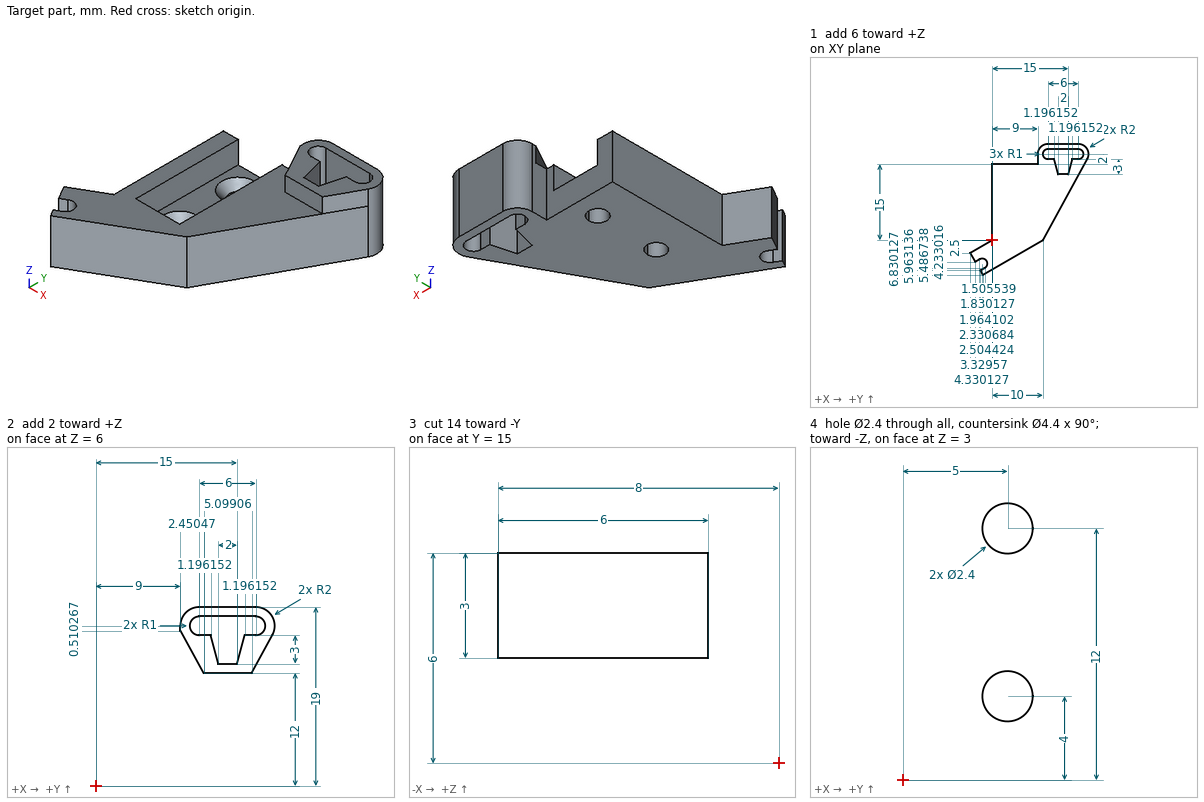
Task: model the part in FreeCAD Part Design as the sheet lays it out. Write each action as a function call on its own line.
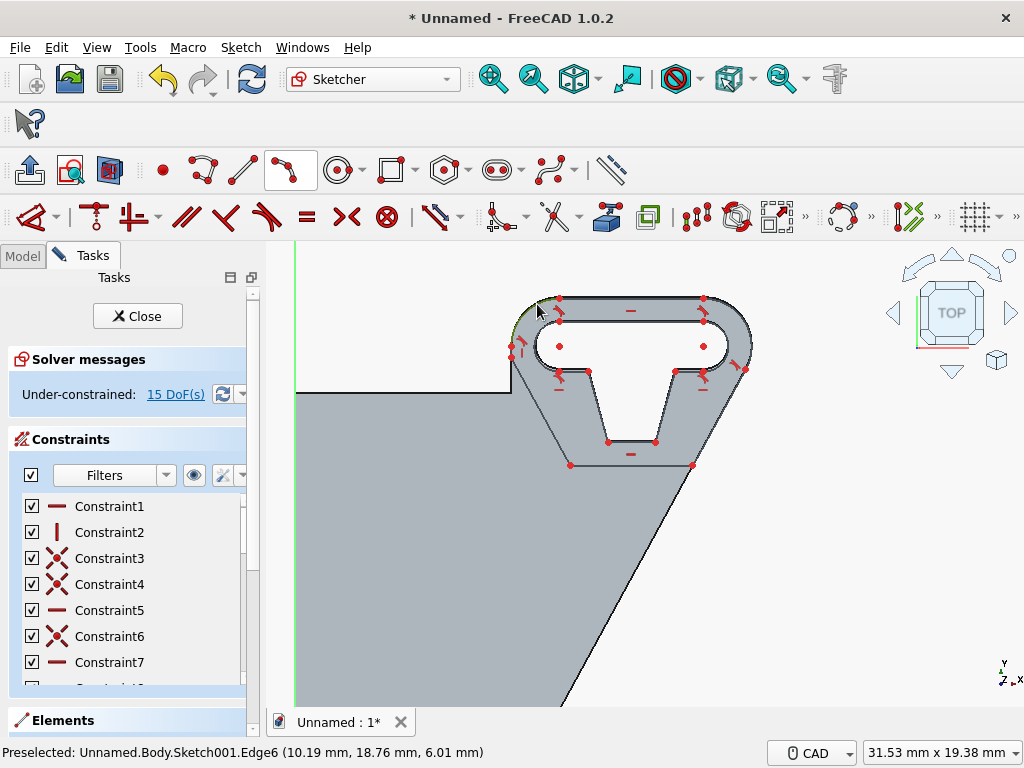
click(751, 341)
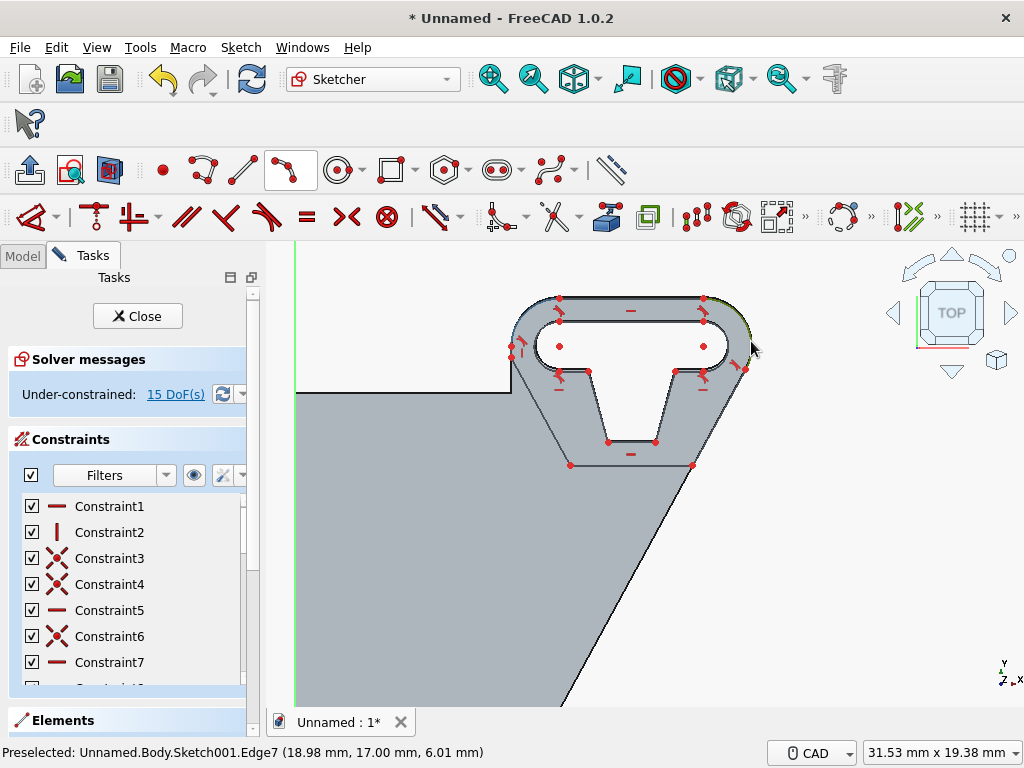
key(e)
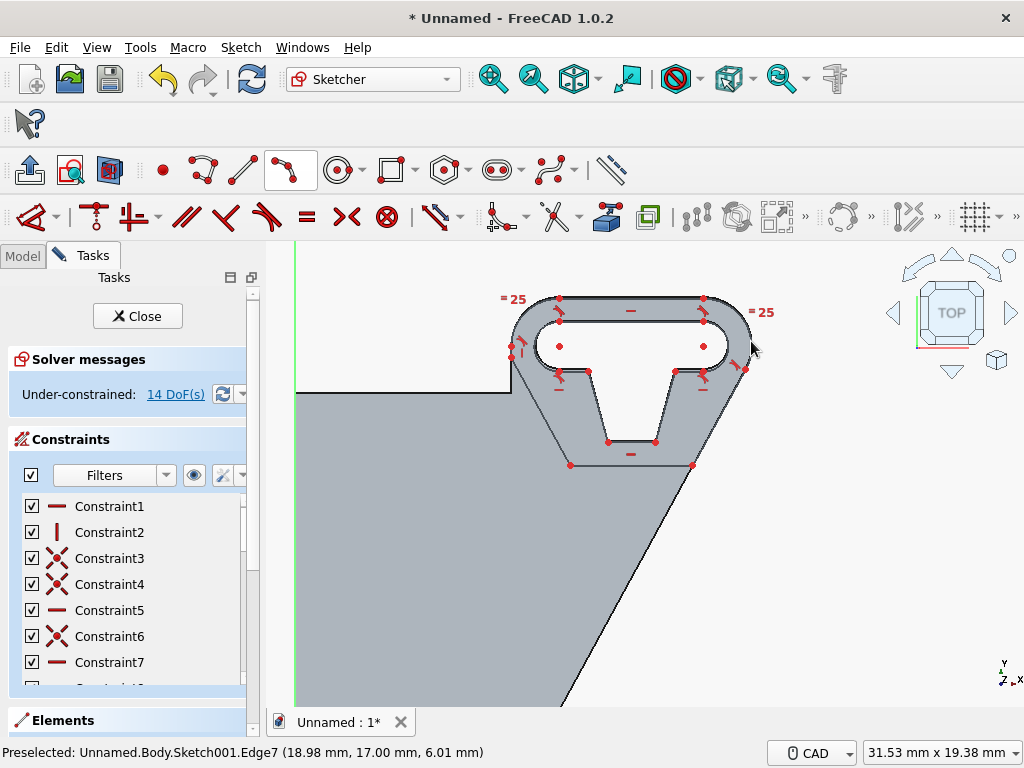
key(d)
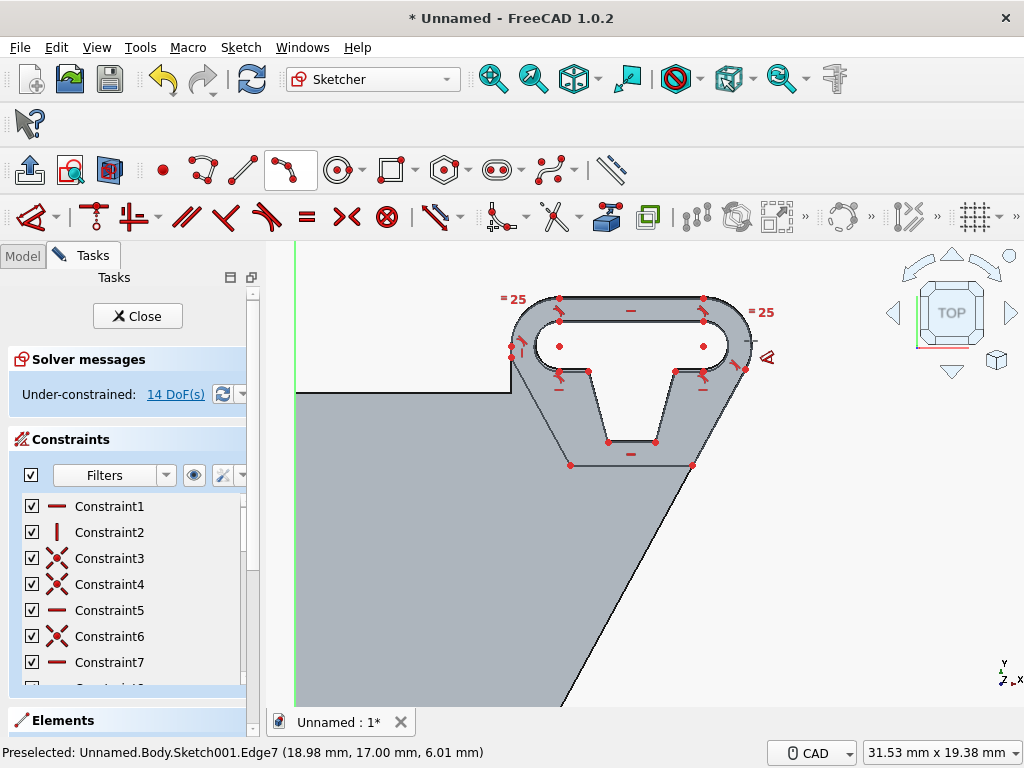
click(537, 304)
click(522, 276)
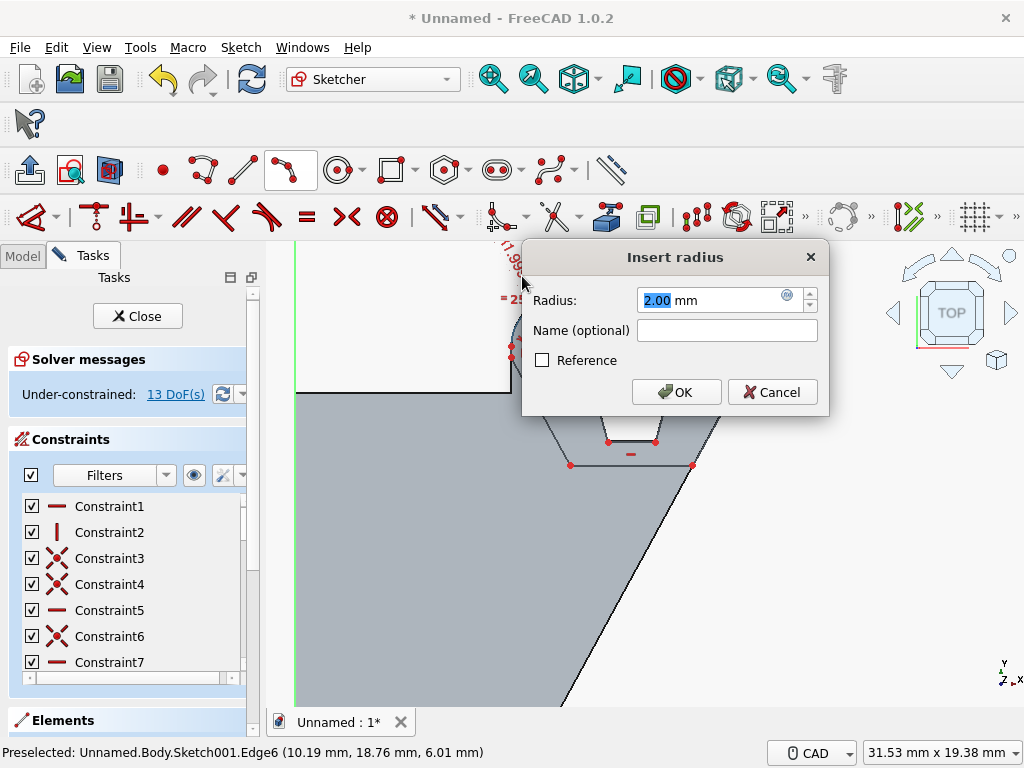
text(2)
key(Return)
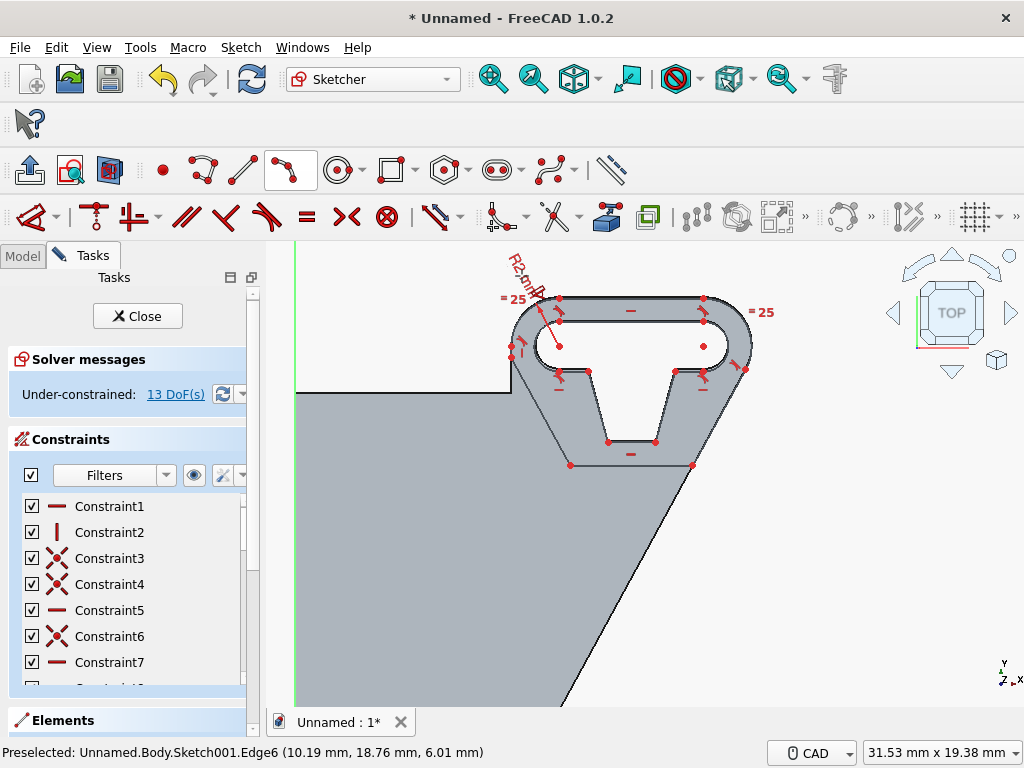
scroll(724, 361, up, 3)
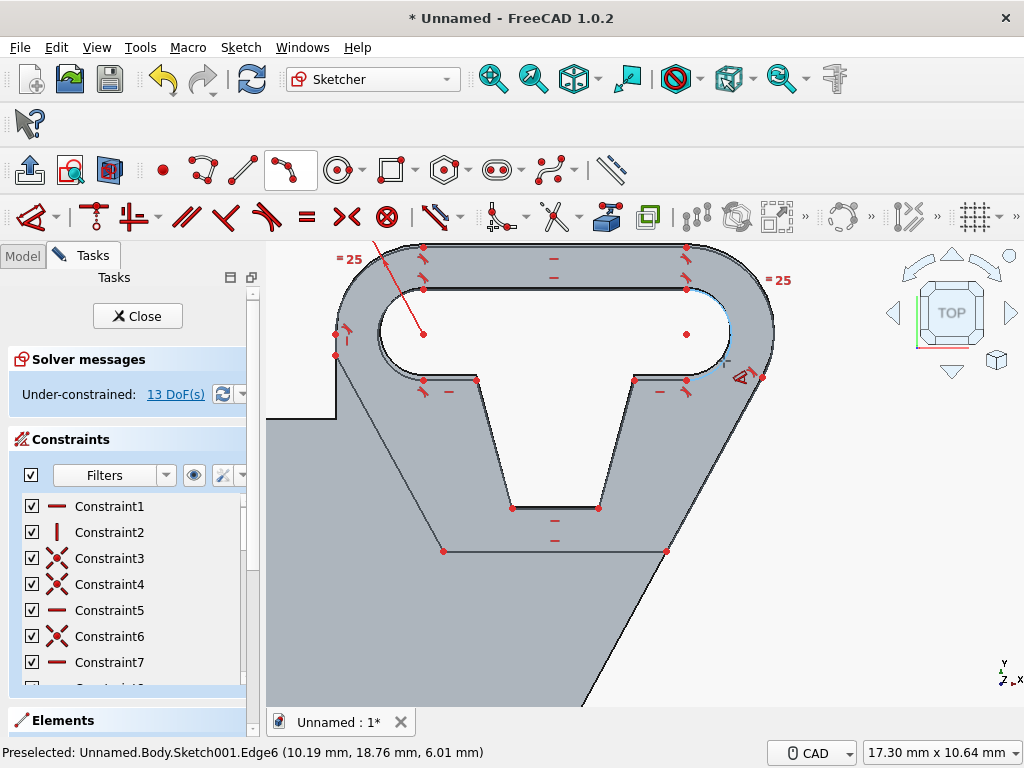
click(723, 362)
click(719, 405)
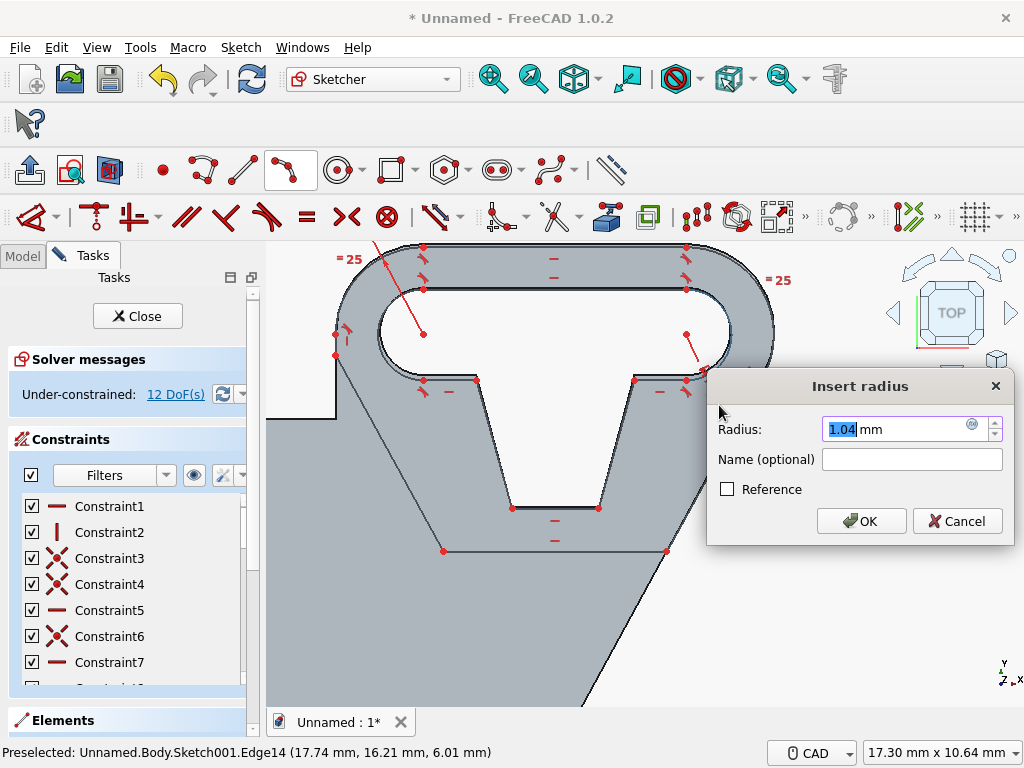
text(1)
key(Return)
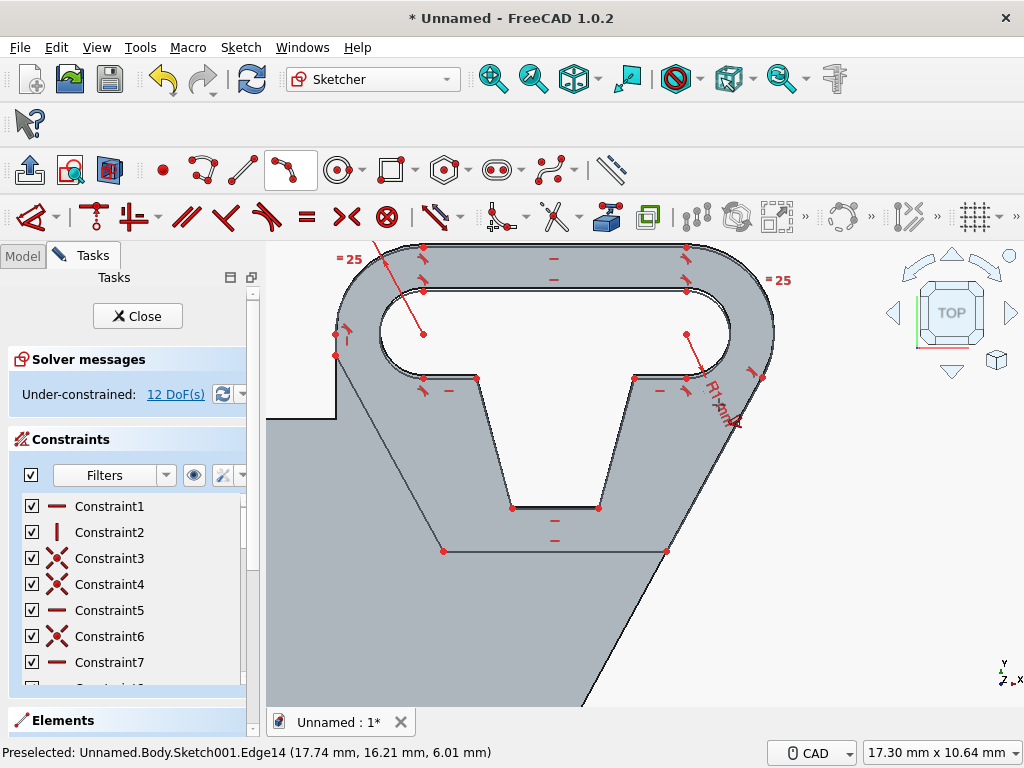
scroll(707, 366, down, 5)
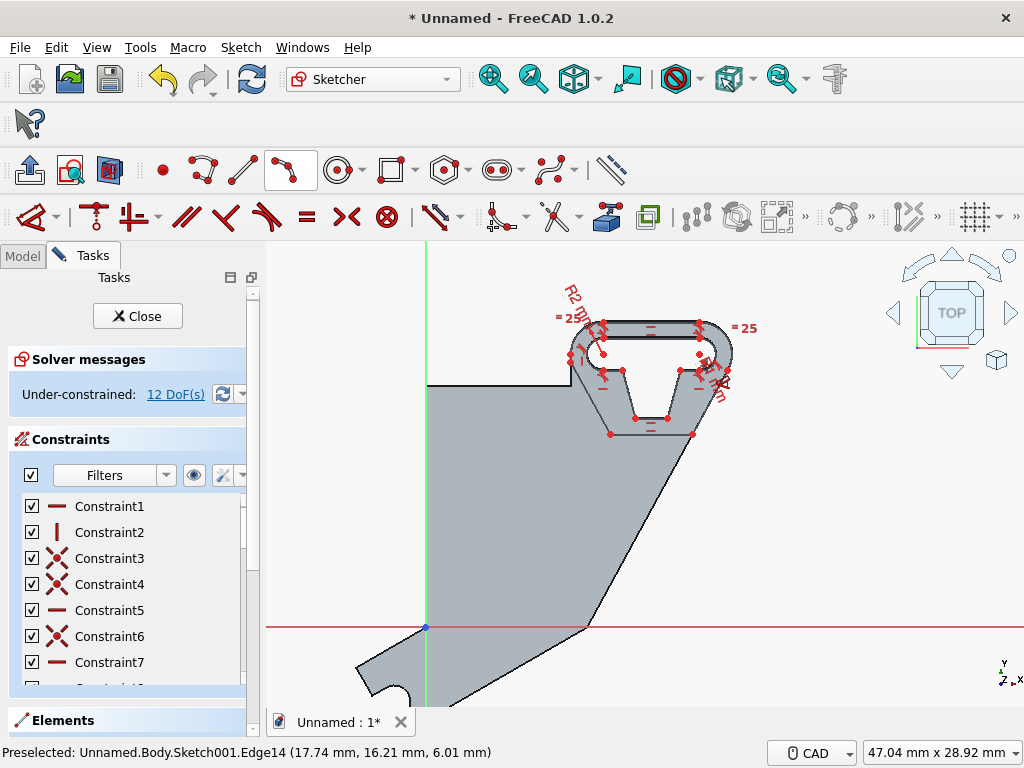
click(671, 323)
click(651, 289)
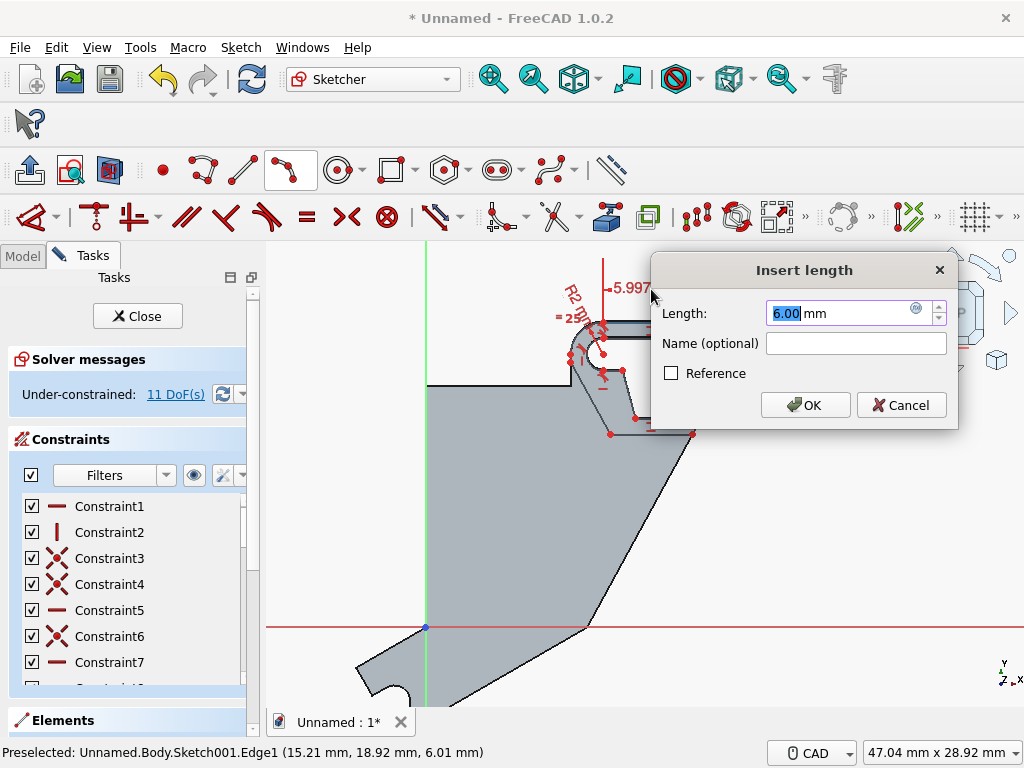
text(6)
key(Return)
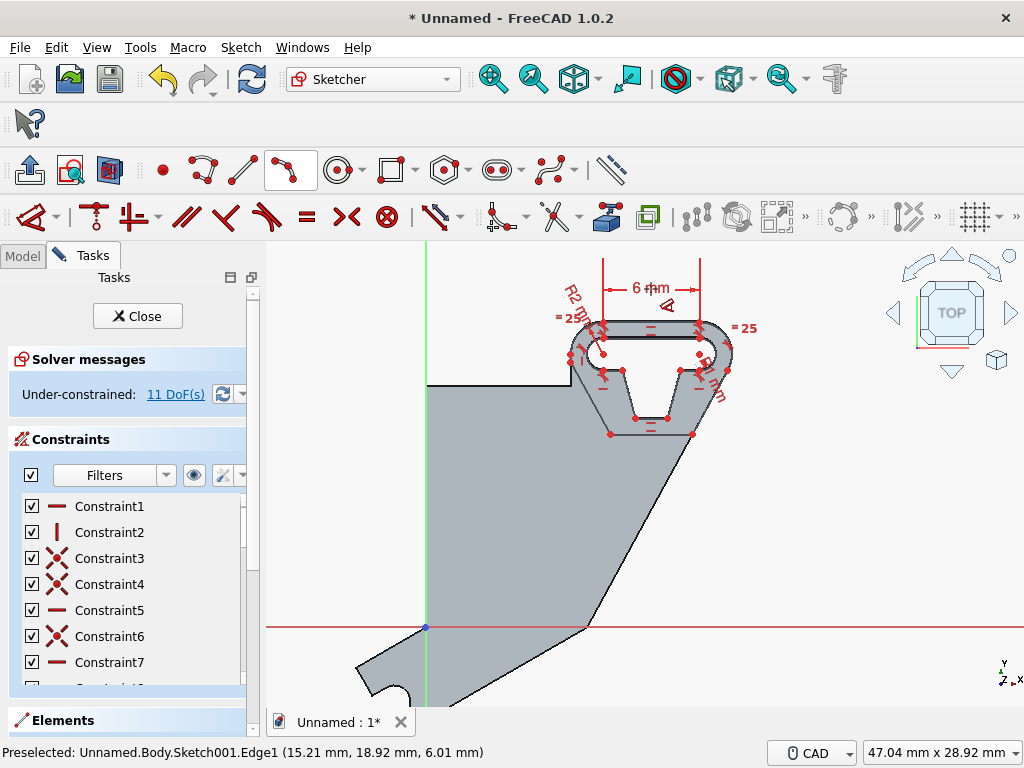
scroll(658, 419, up, 2)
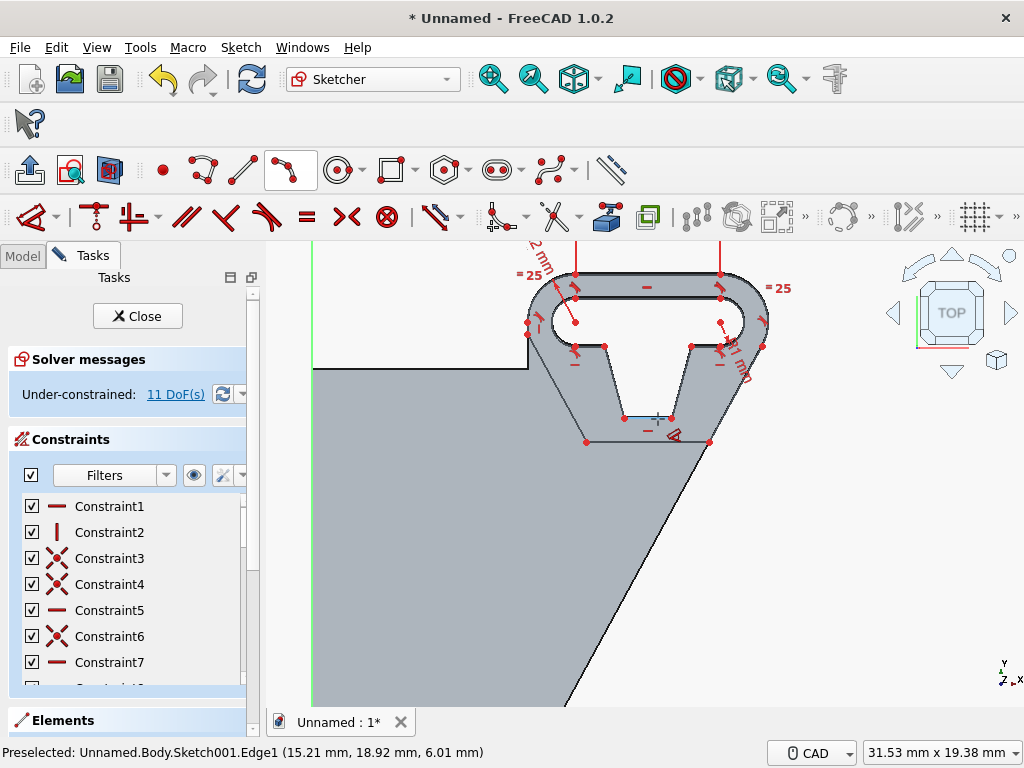
click(658, 418)
click(648, 384)